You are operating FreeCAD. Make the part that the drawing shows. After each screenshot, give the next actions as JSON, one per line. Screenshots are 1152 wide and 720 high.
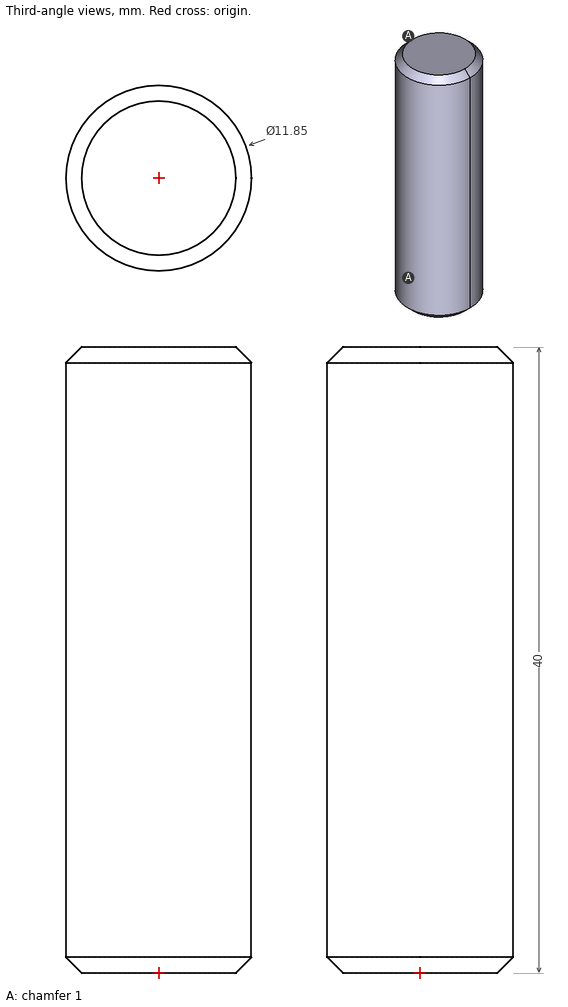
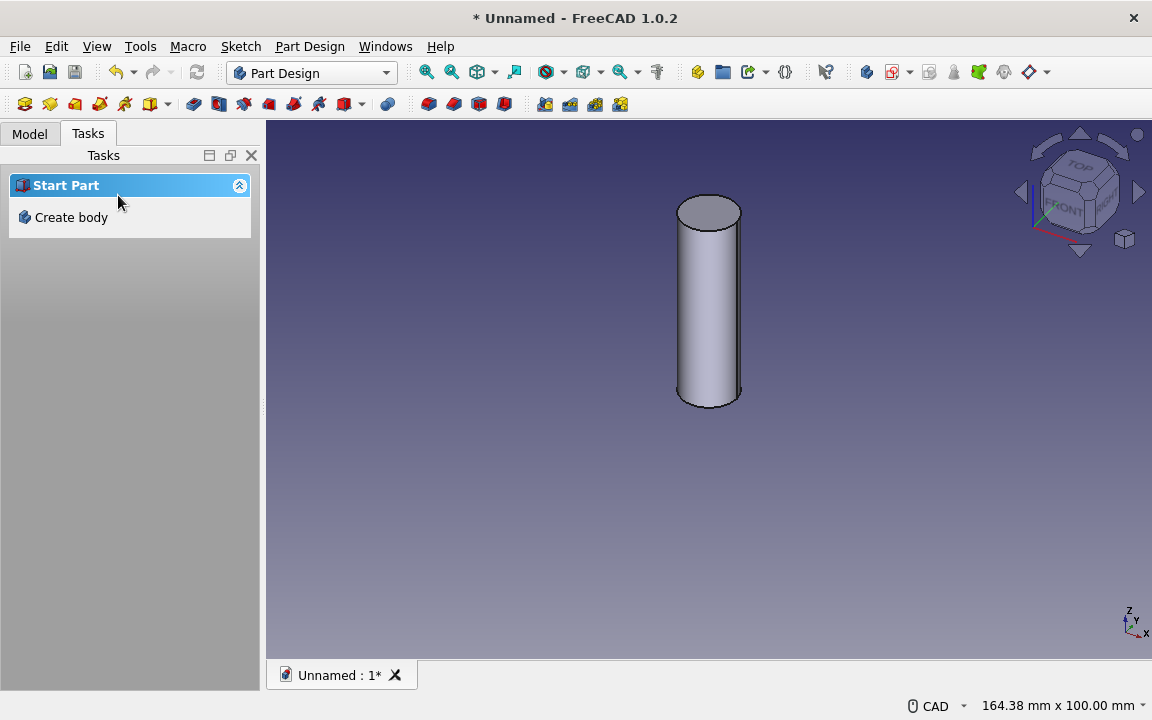
{"action": "left_click", "coordinate": [427, 72]}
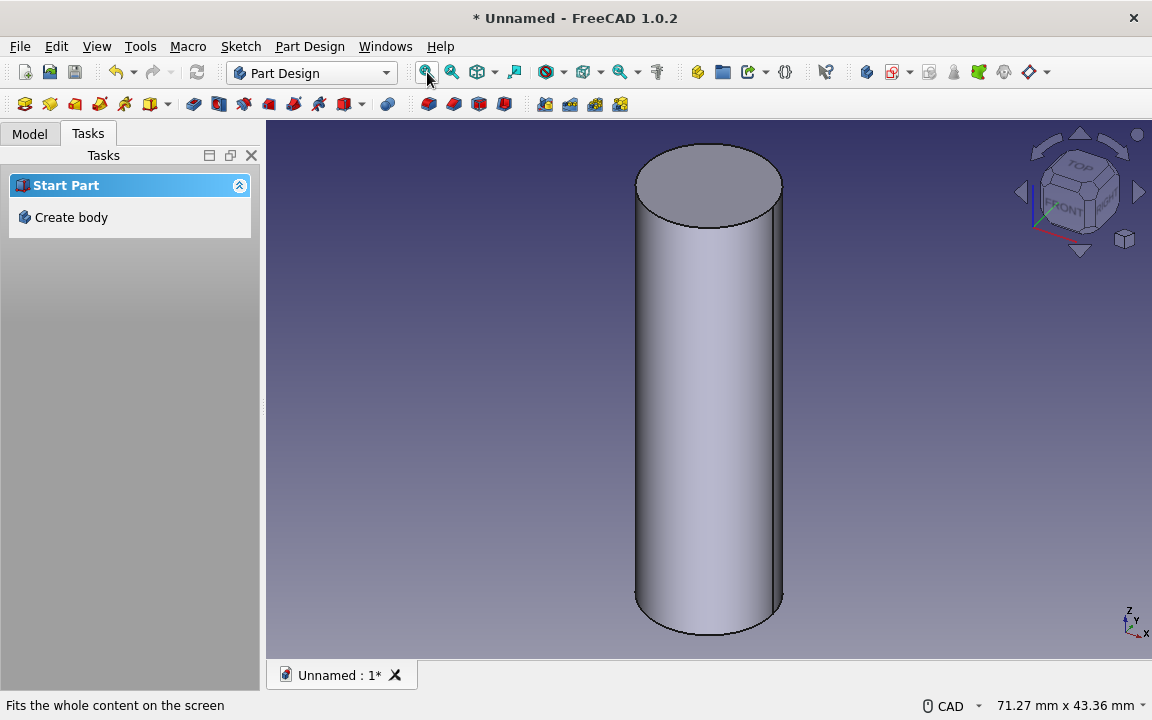
{"action": "left_click", "coordinate": [636, 189]}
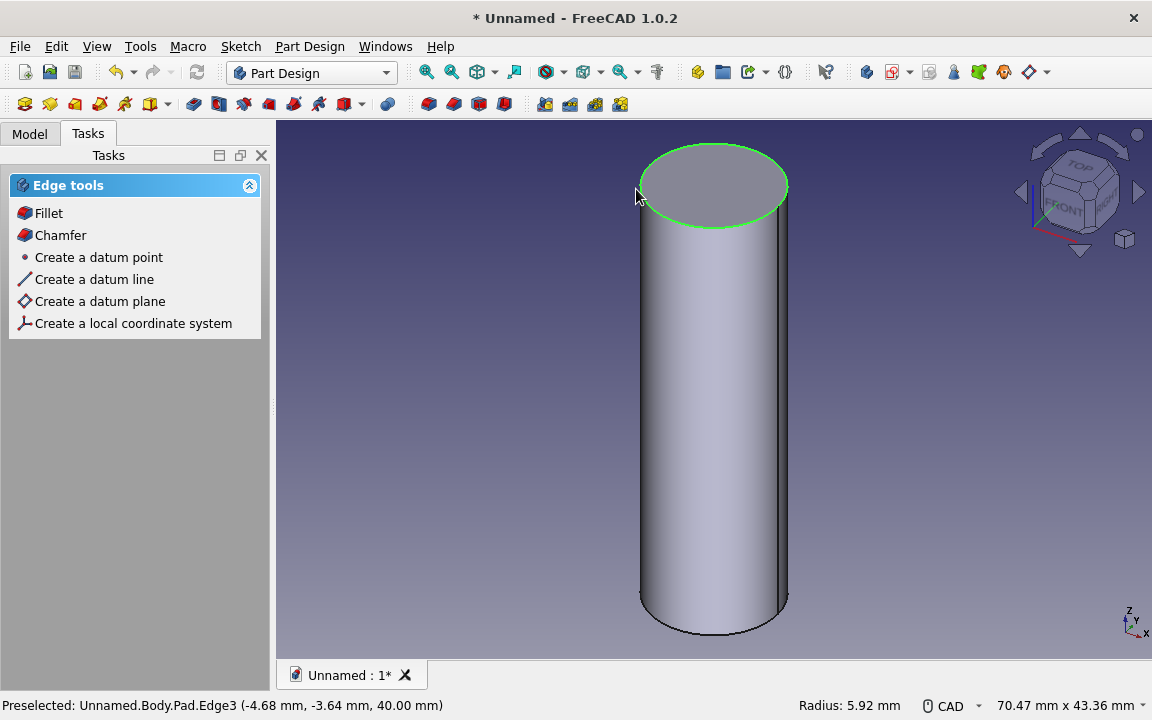
{"action": "key", "text": "0"}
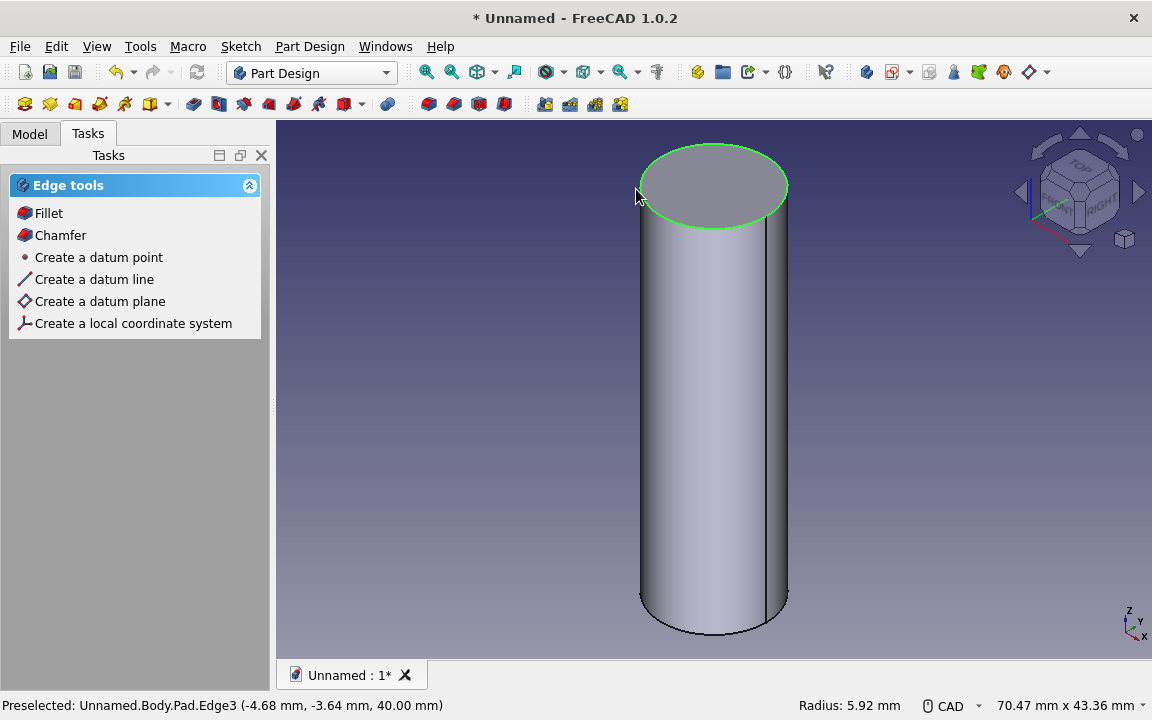
{"action": "left_click", "coordinate": [648, 611], "text": "ctrl"}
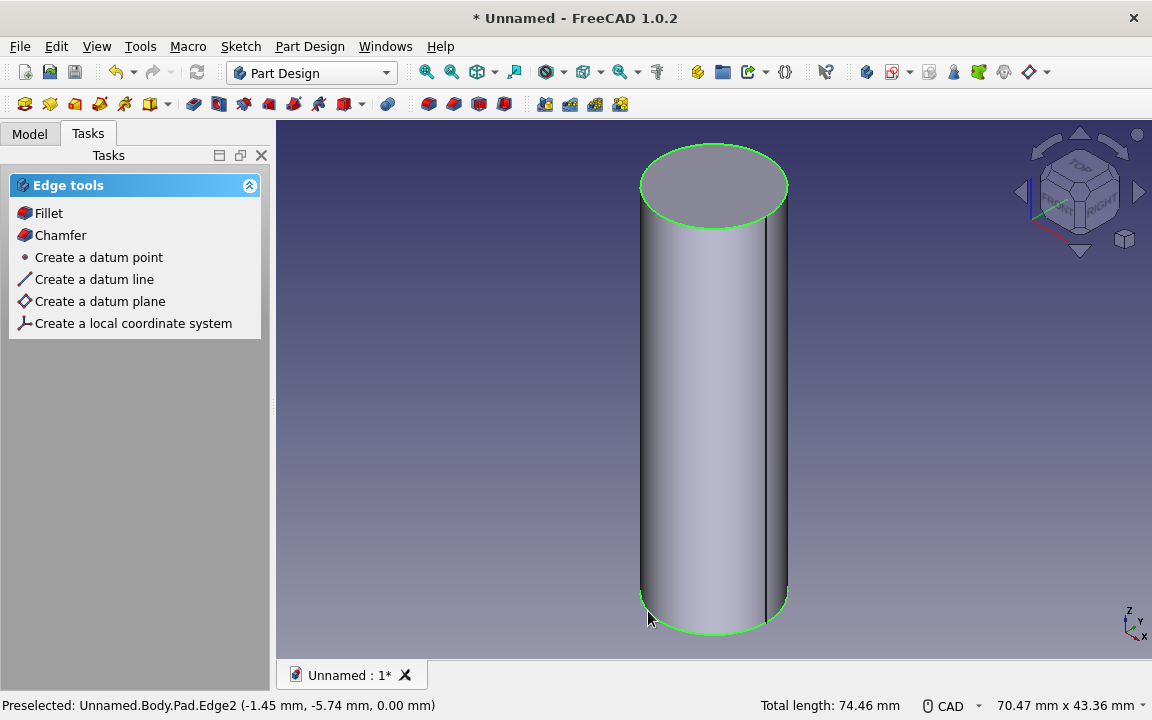
{"action": "left_click", "coordinate": [454, 104]}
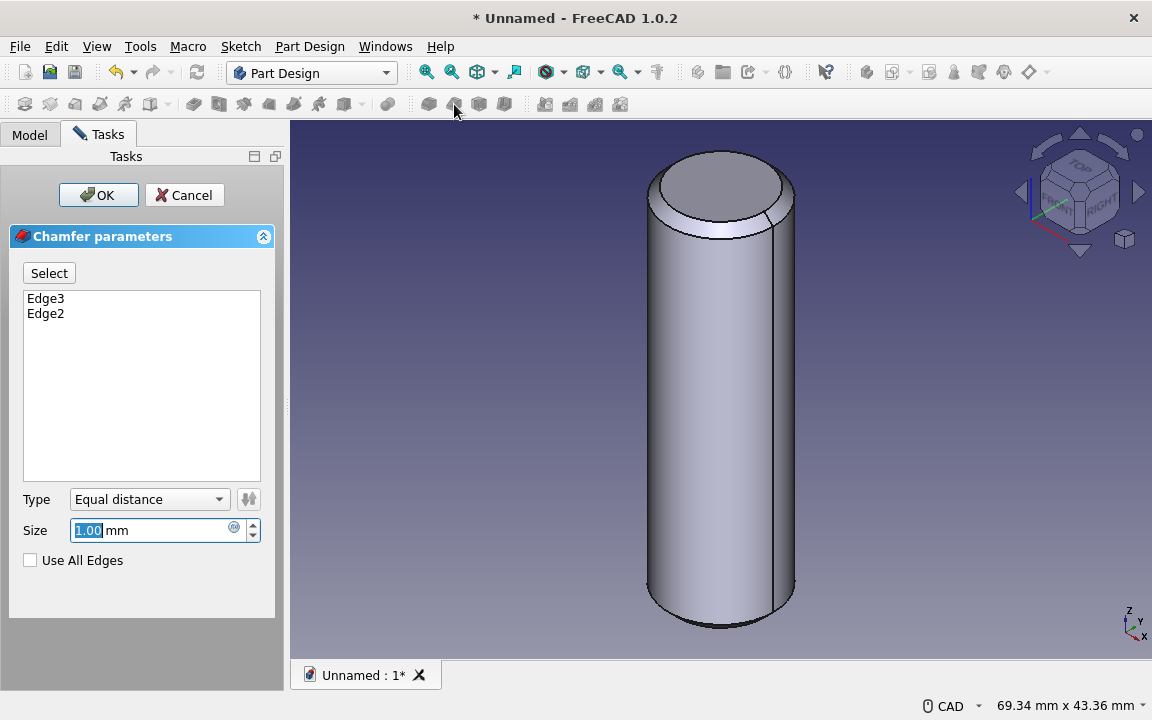
{"action": "type", "text": "1"}
{"action": "key", "text": "Tab"}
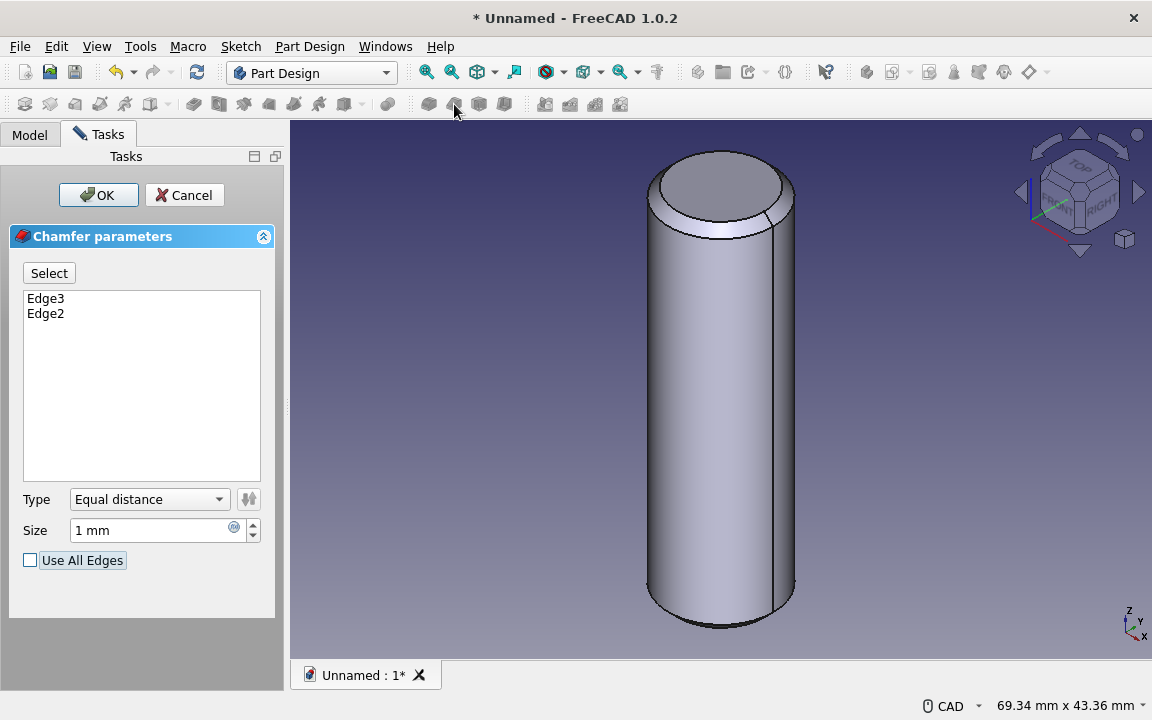
{"action": "left_click", "coordinate": [99, 195]}